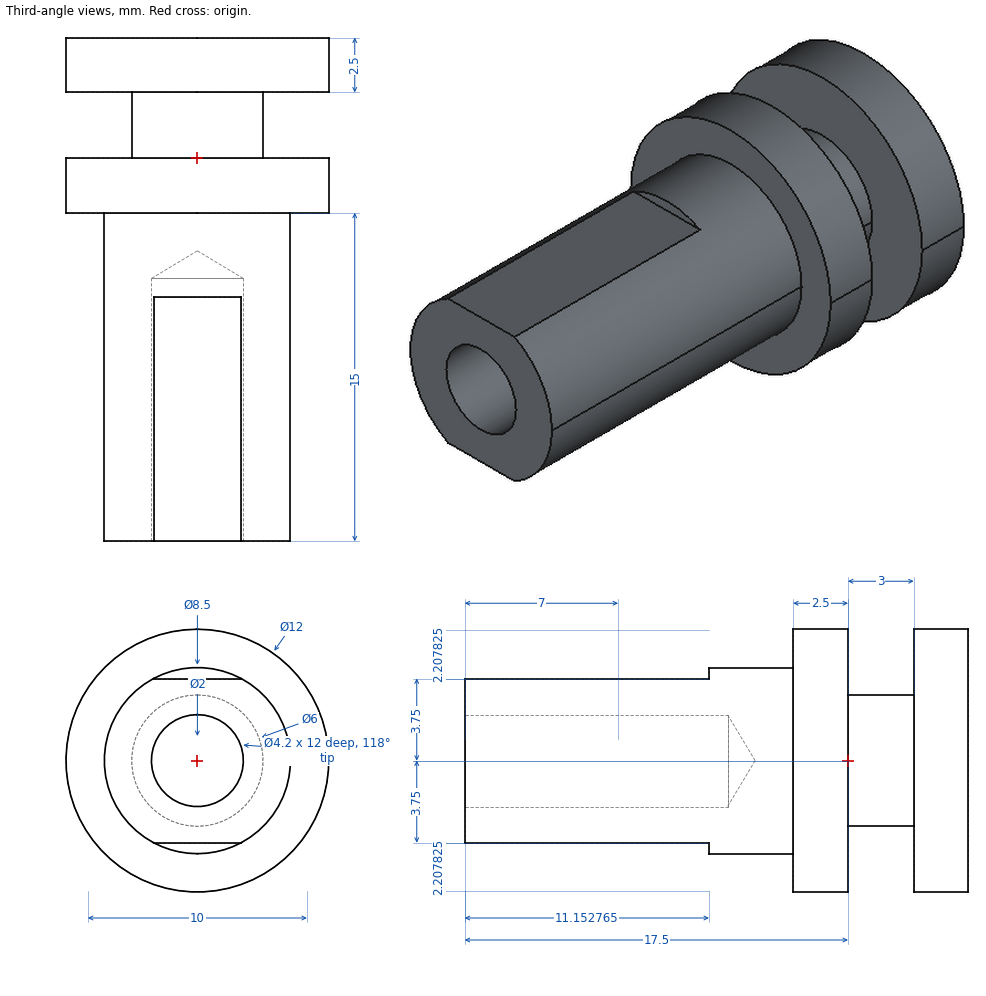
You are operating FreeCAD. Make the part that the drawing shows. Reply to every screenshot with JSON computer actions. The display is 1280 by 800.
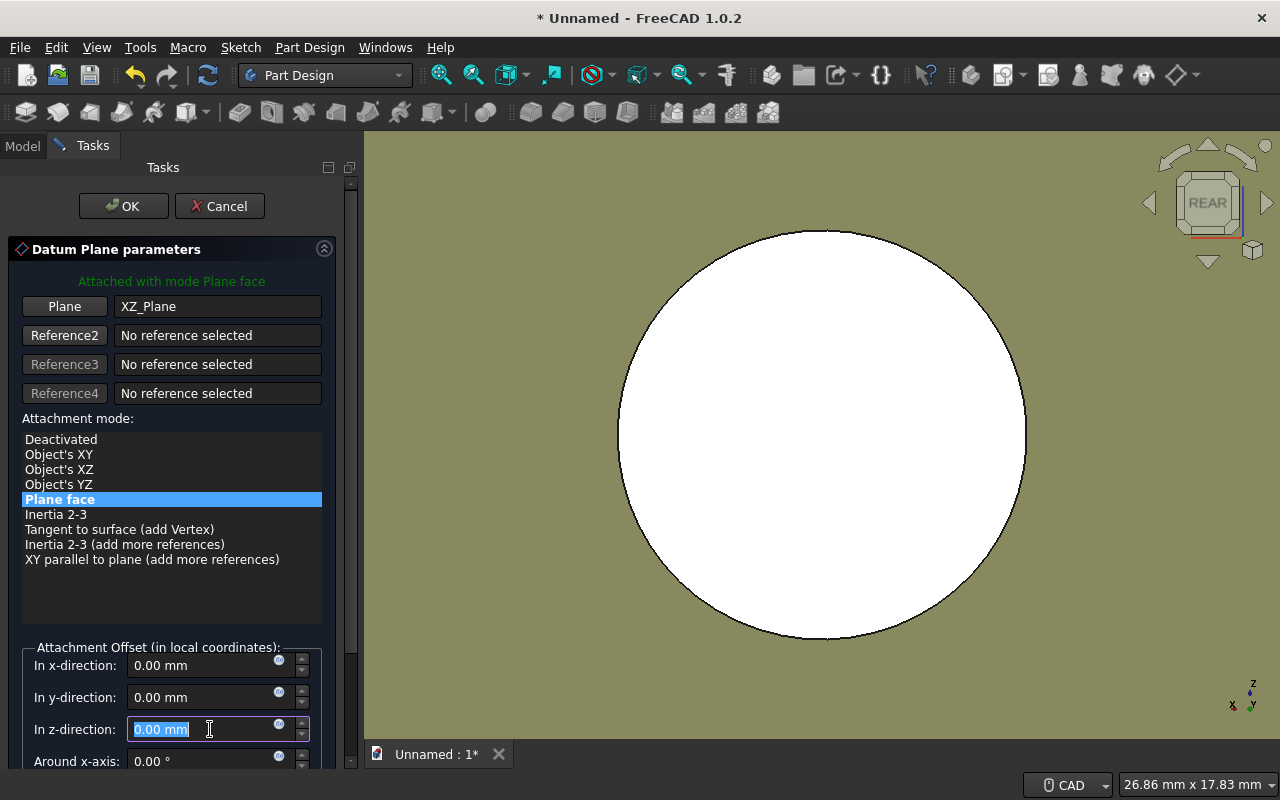
{"action": "type", "text": "2.5"}
{"action": "key", "text": "Tab"}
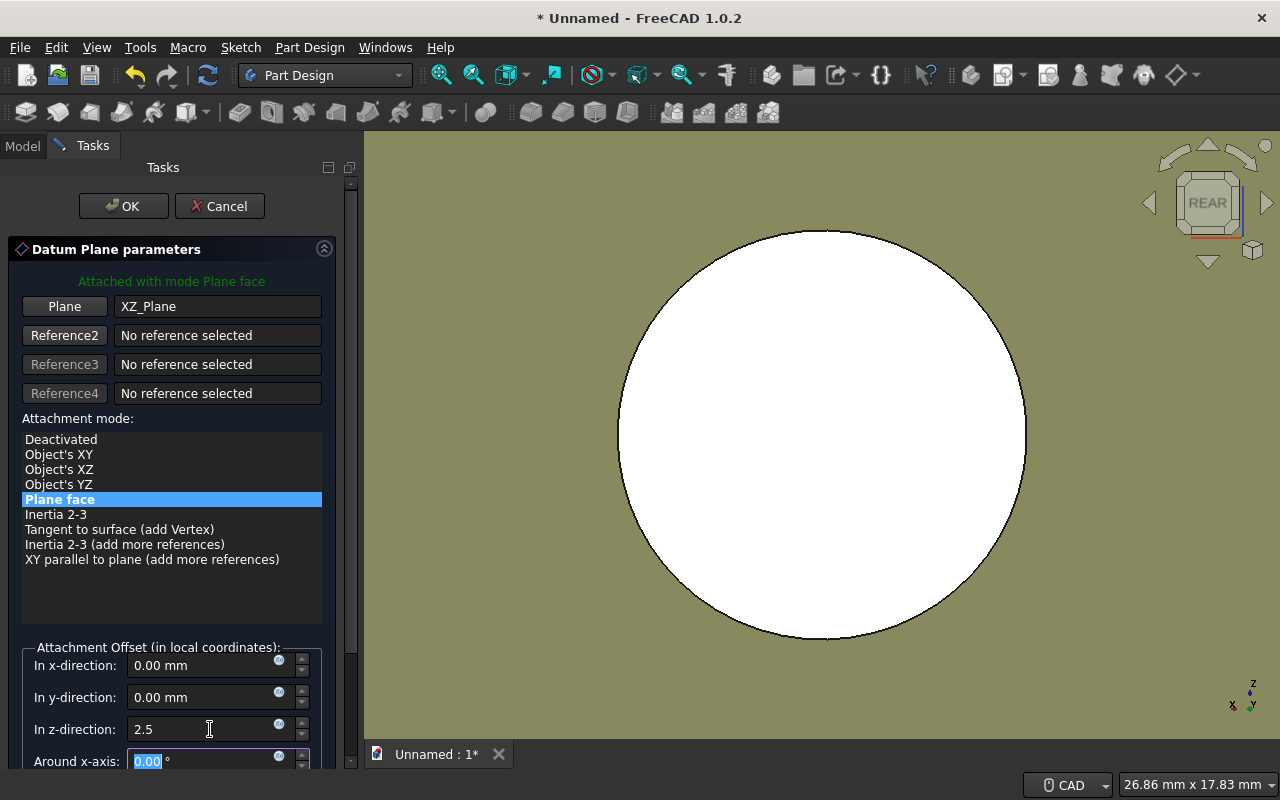
{"action": "left_click", "coordinate": [124, 206]}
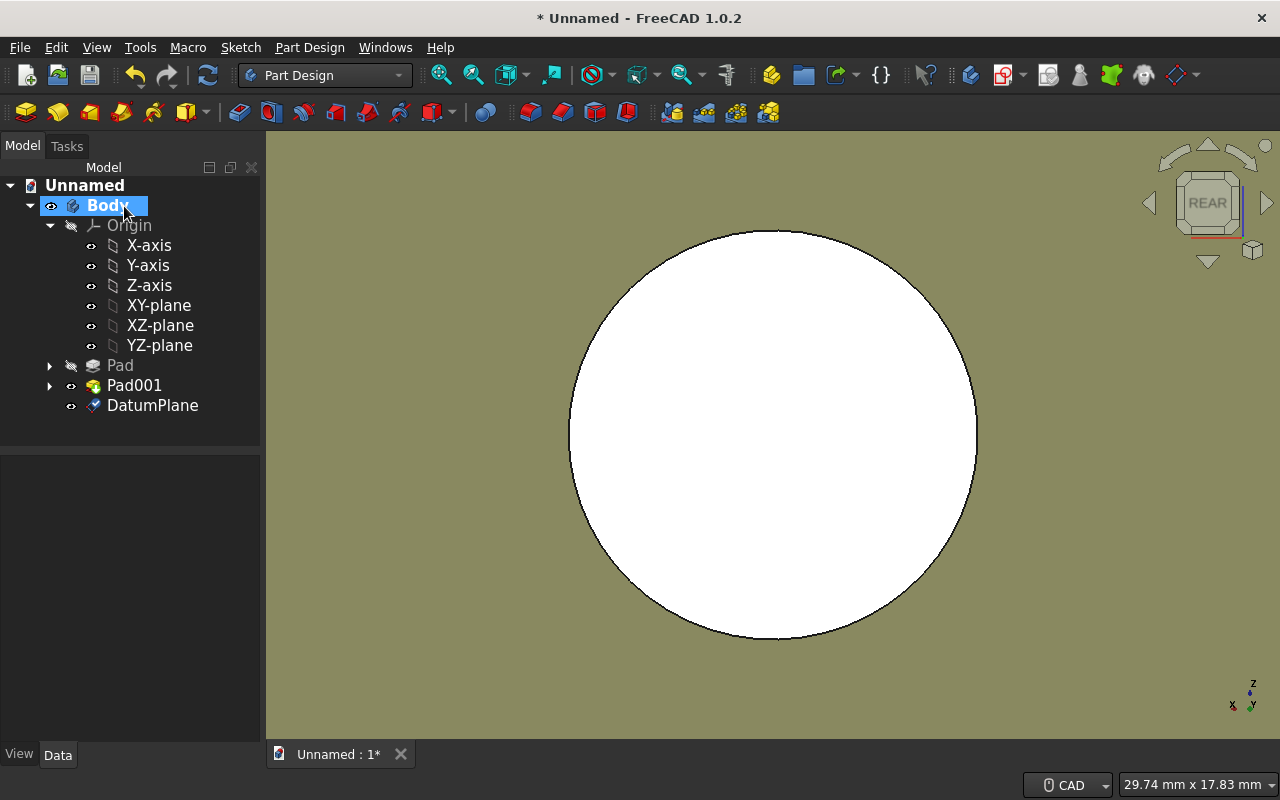
{"action": "left_click", "coordinate": [116, 406]}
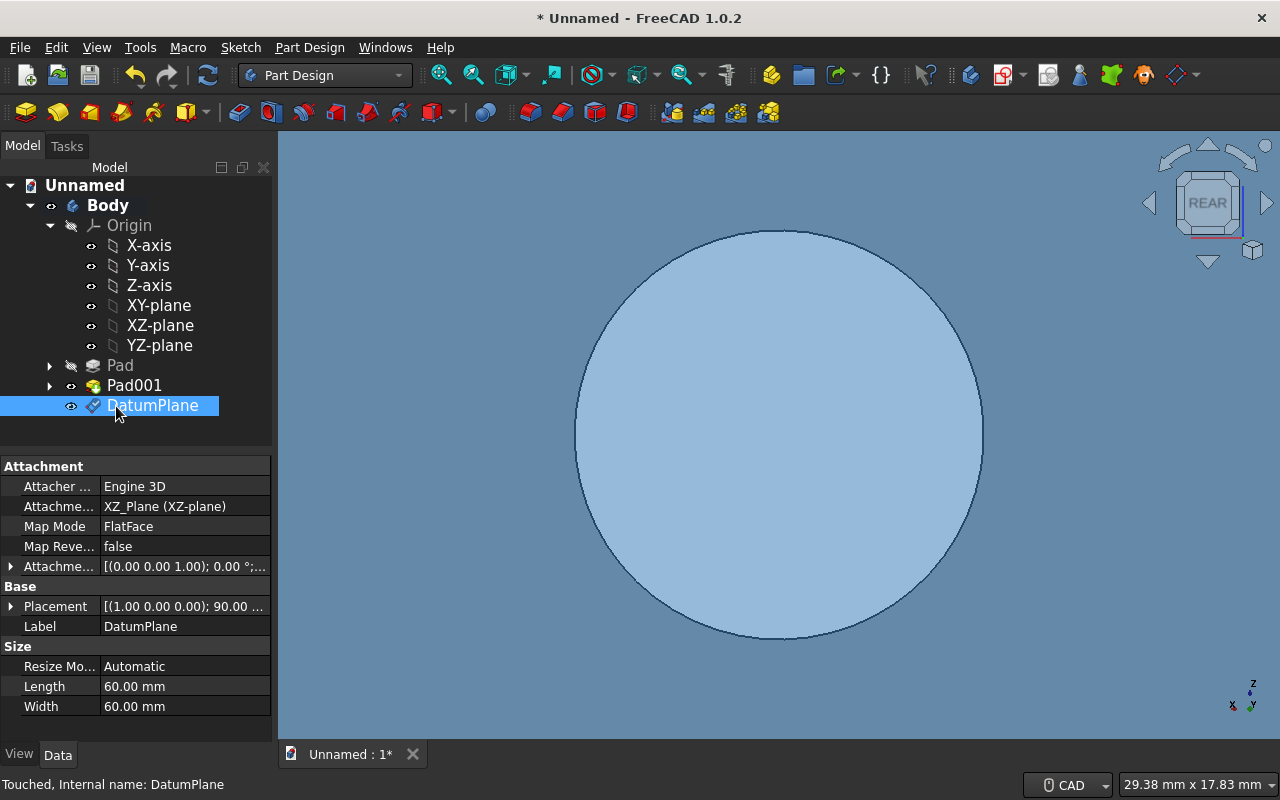
{"action": "left_click", "coordinate": [1004, 76]}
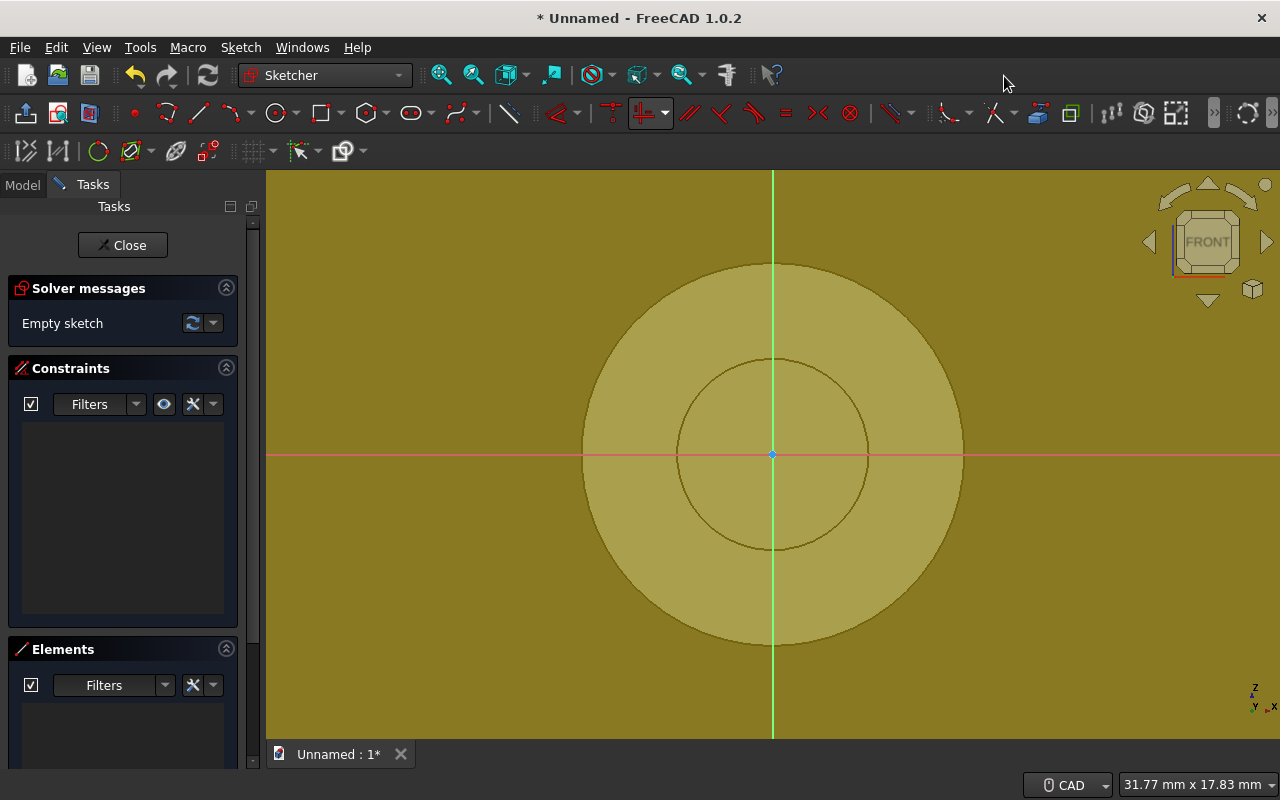
{"action": "key", "text": "g c"}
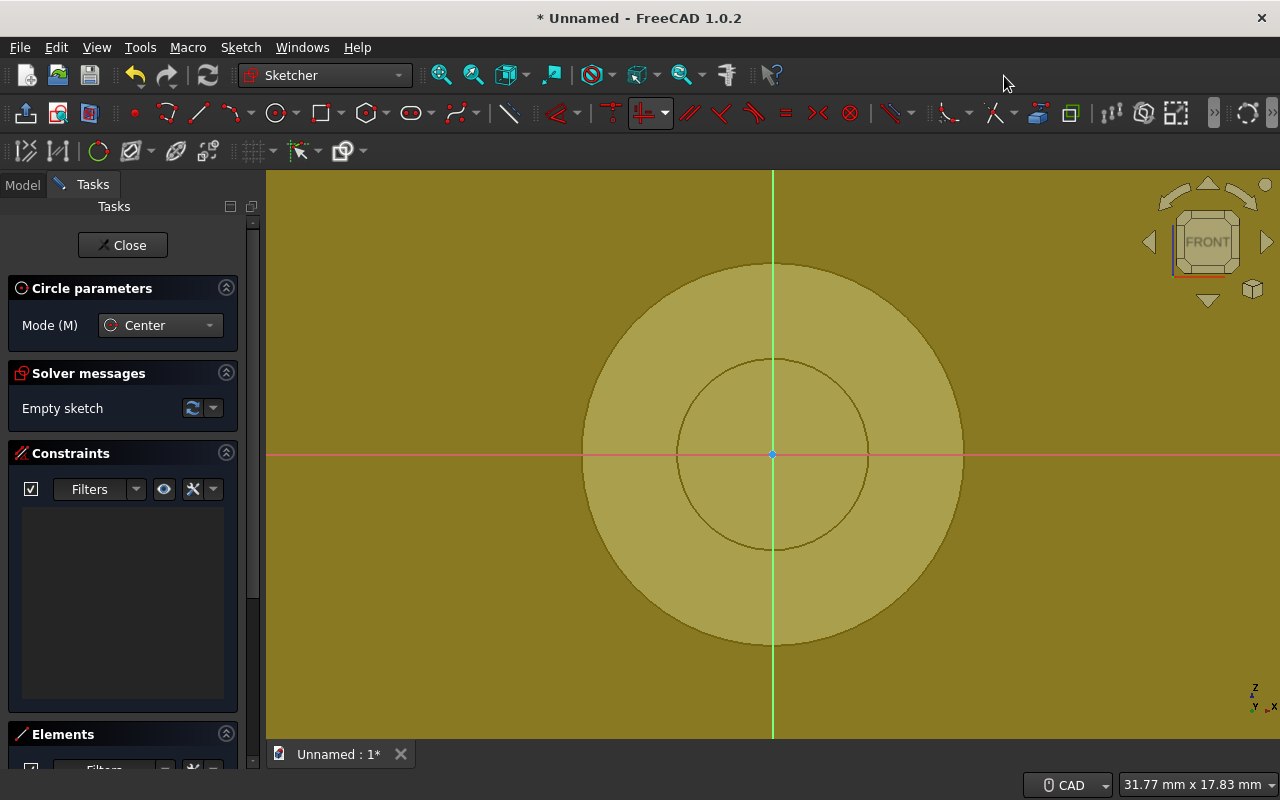
{"action": "left_click", "coordinate": [773, 455]}
{"action": "mouse_move", "coordinate": [908, 319]}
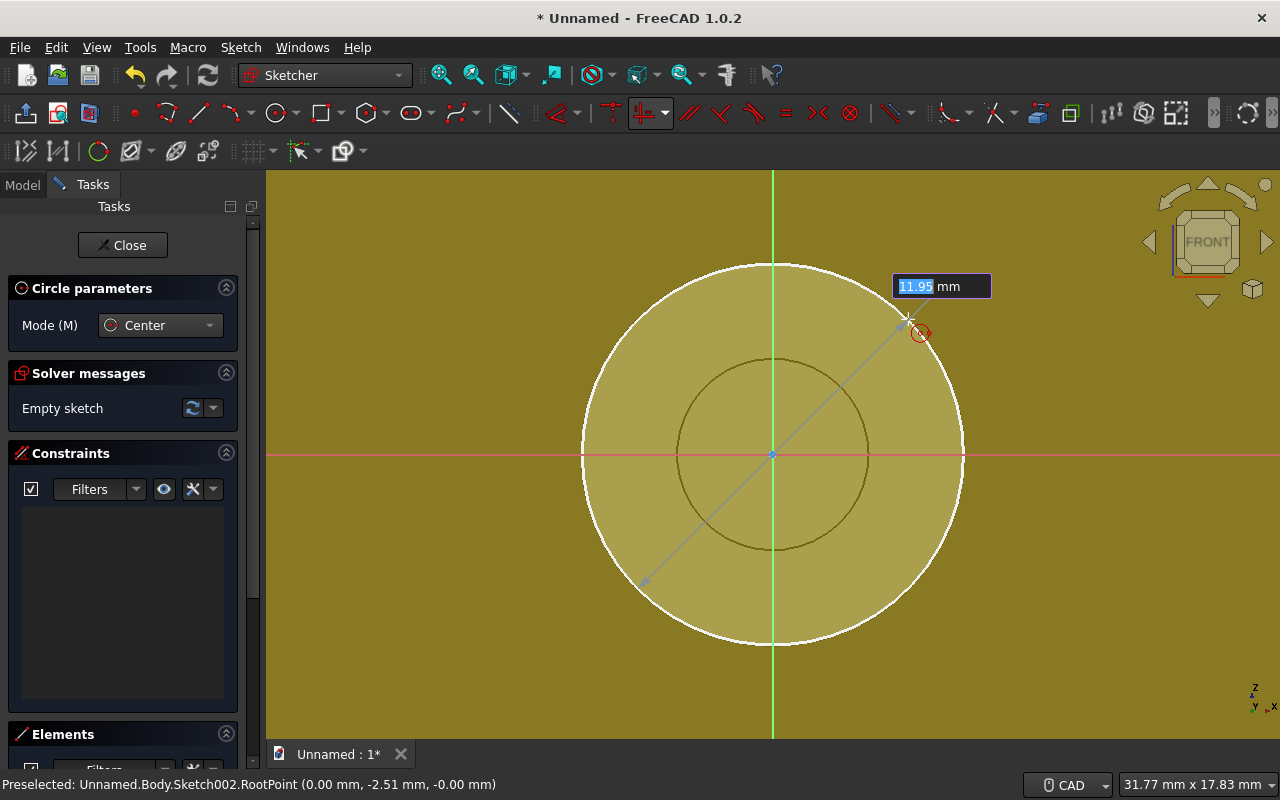
{"action": "type", "text": "12"}
{"action": "key", "text": "Return"}
{"action": "key", "text": "Escape"}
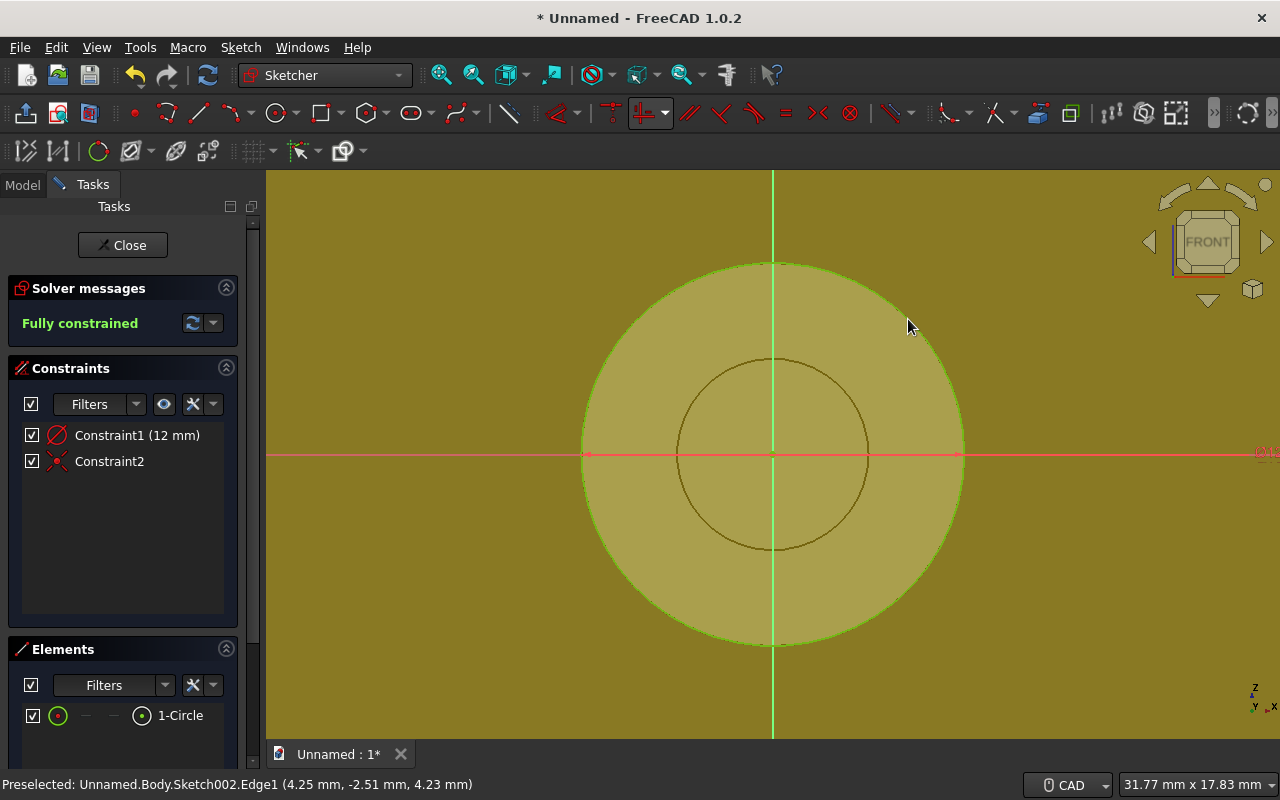
{"action": "left_click", "coordinate": [123, 245]}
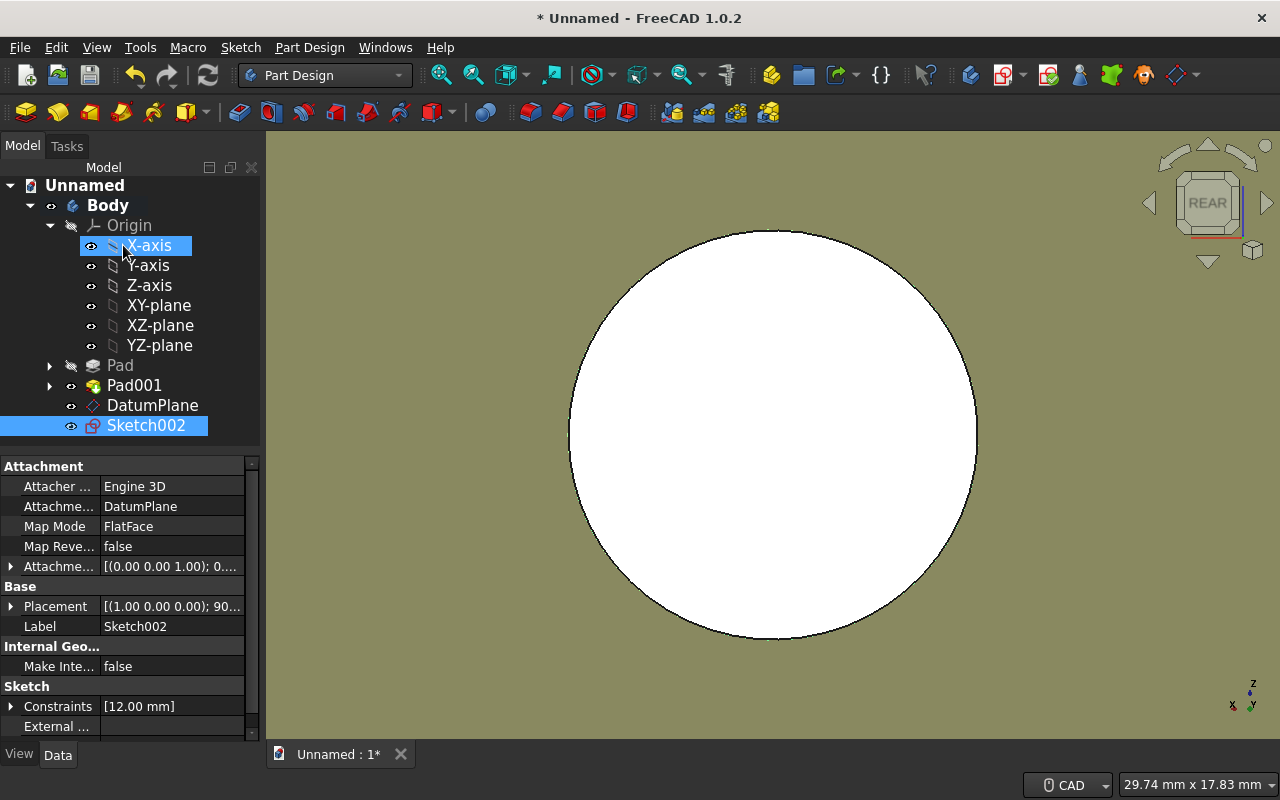
{"action": "left_click", "coordinate": [26, 112]}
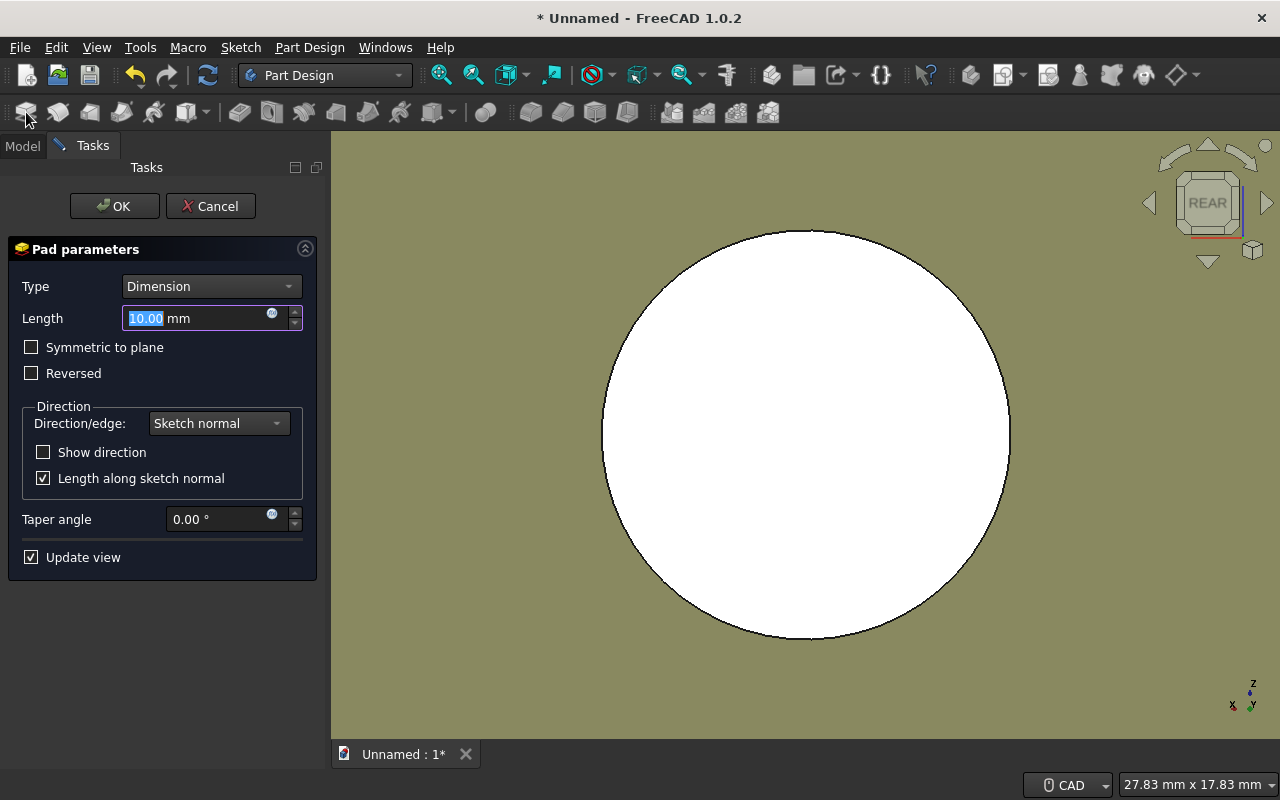
{"action": "type", "text": "2.5"}
{"action": "key", "text": "Tab"}